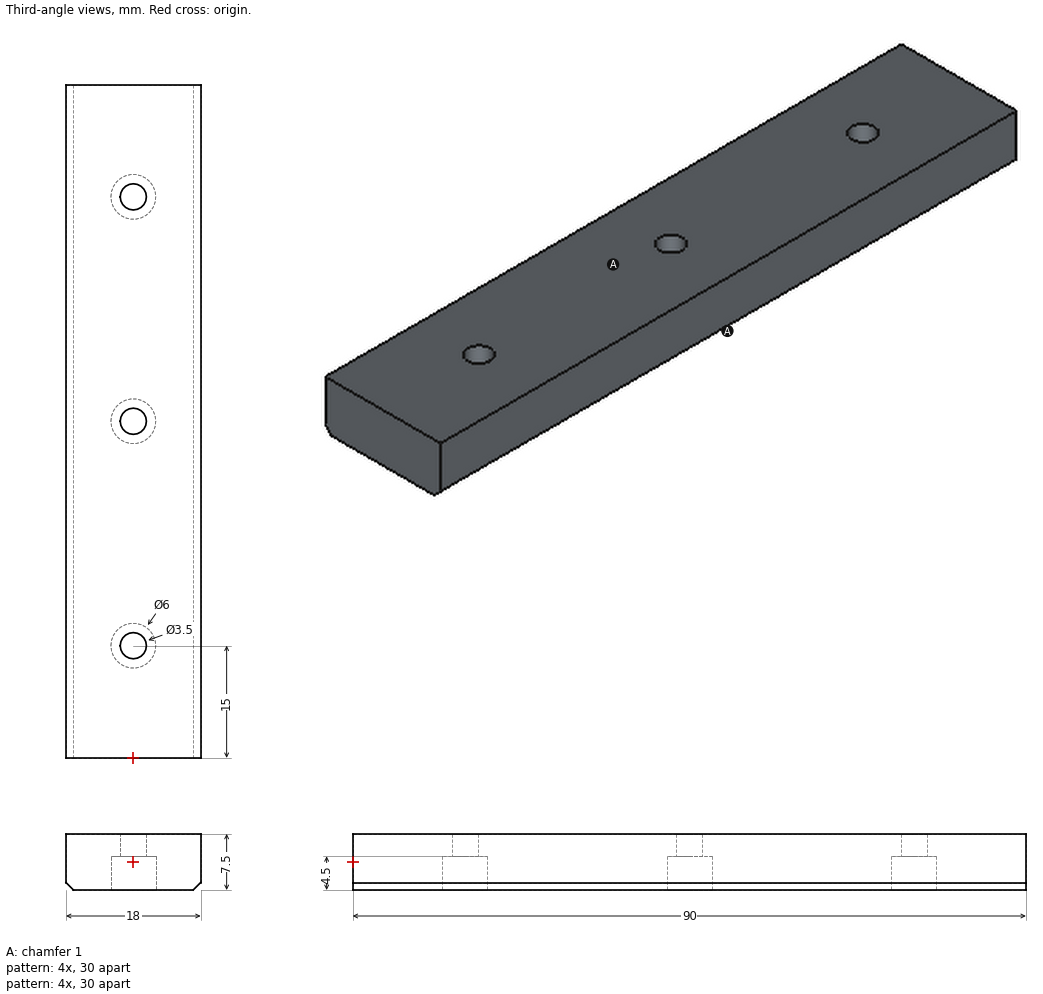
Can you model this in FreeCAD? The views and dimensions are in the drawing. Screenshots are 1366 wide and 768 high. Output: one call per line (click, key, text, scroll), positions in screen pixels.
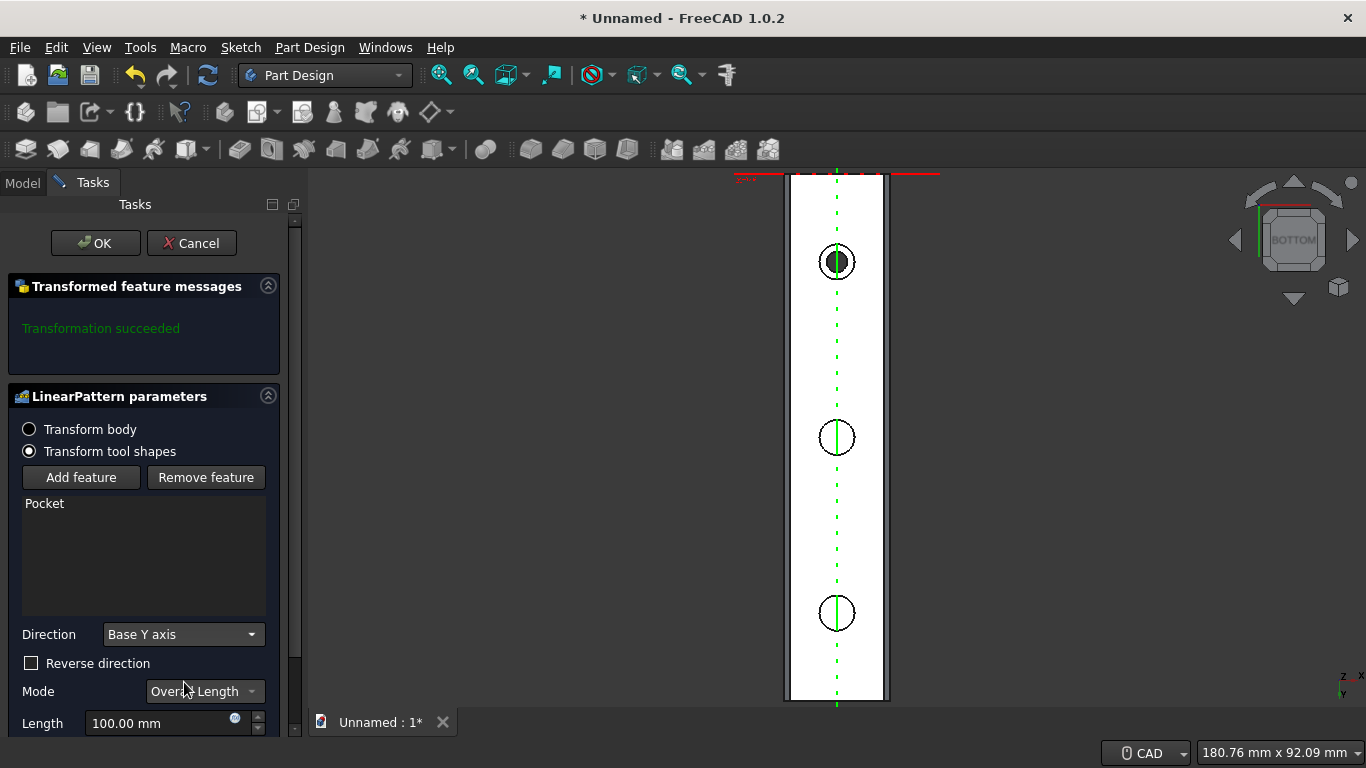
click(206, 692)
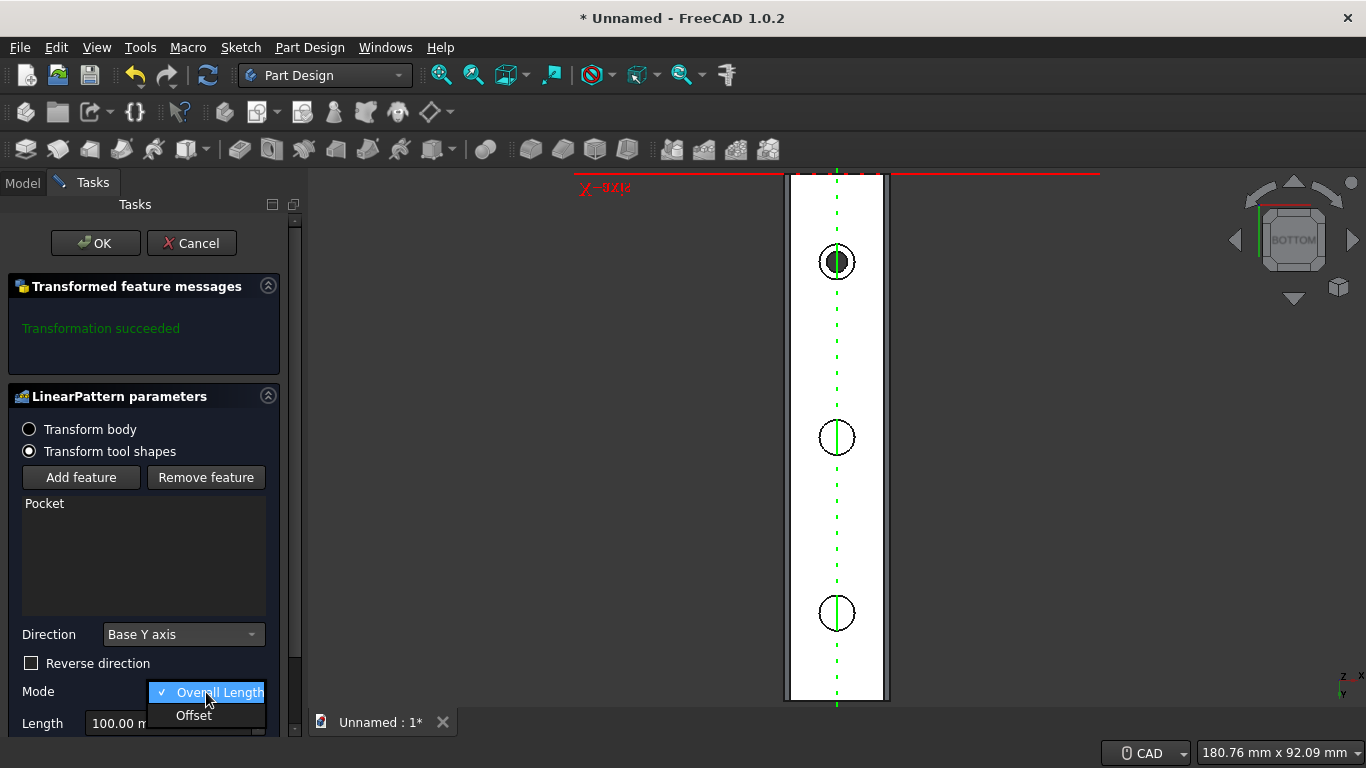
click(206, 716)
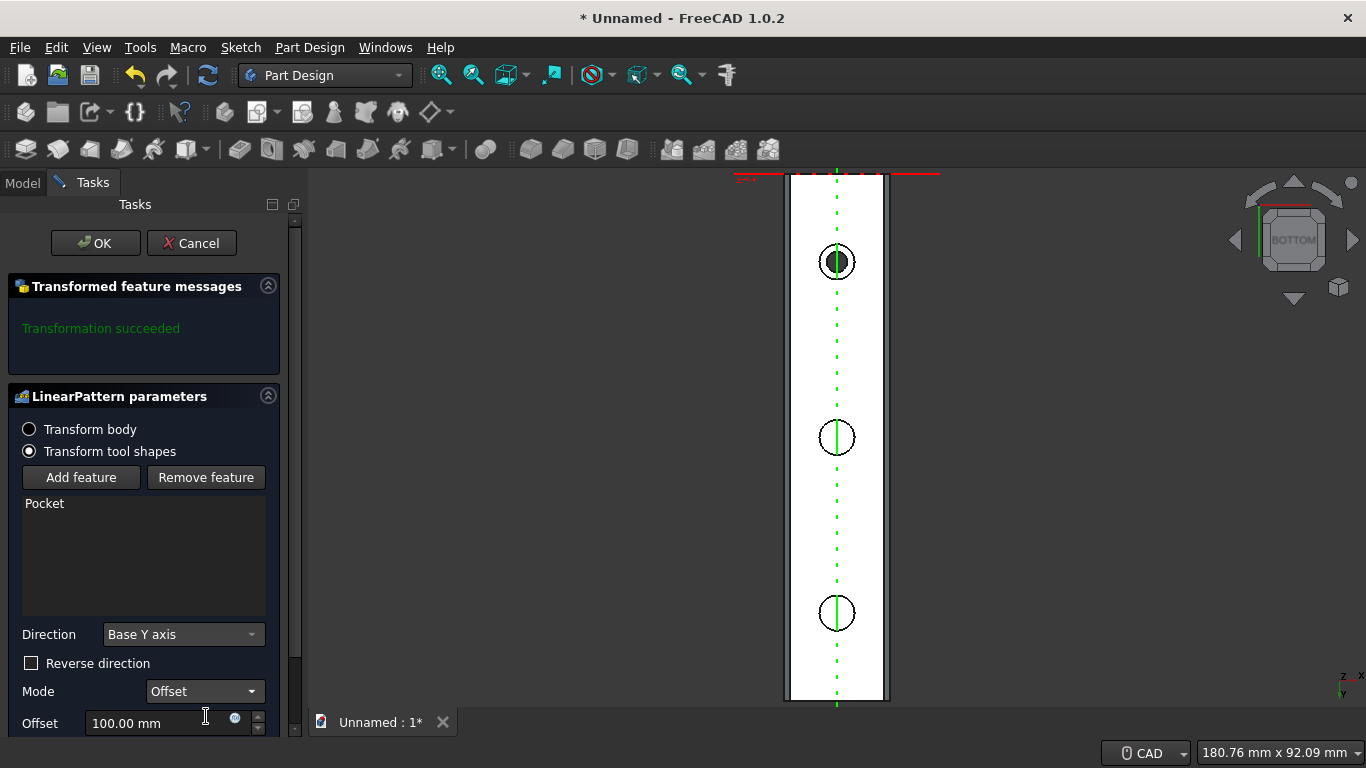
triple_click(168, 723)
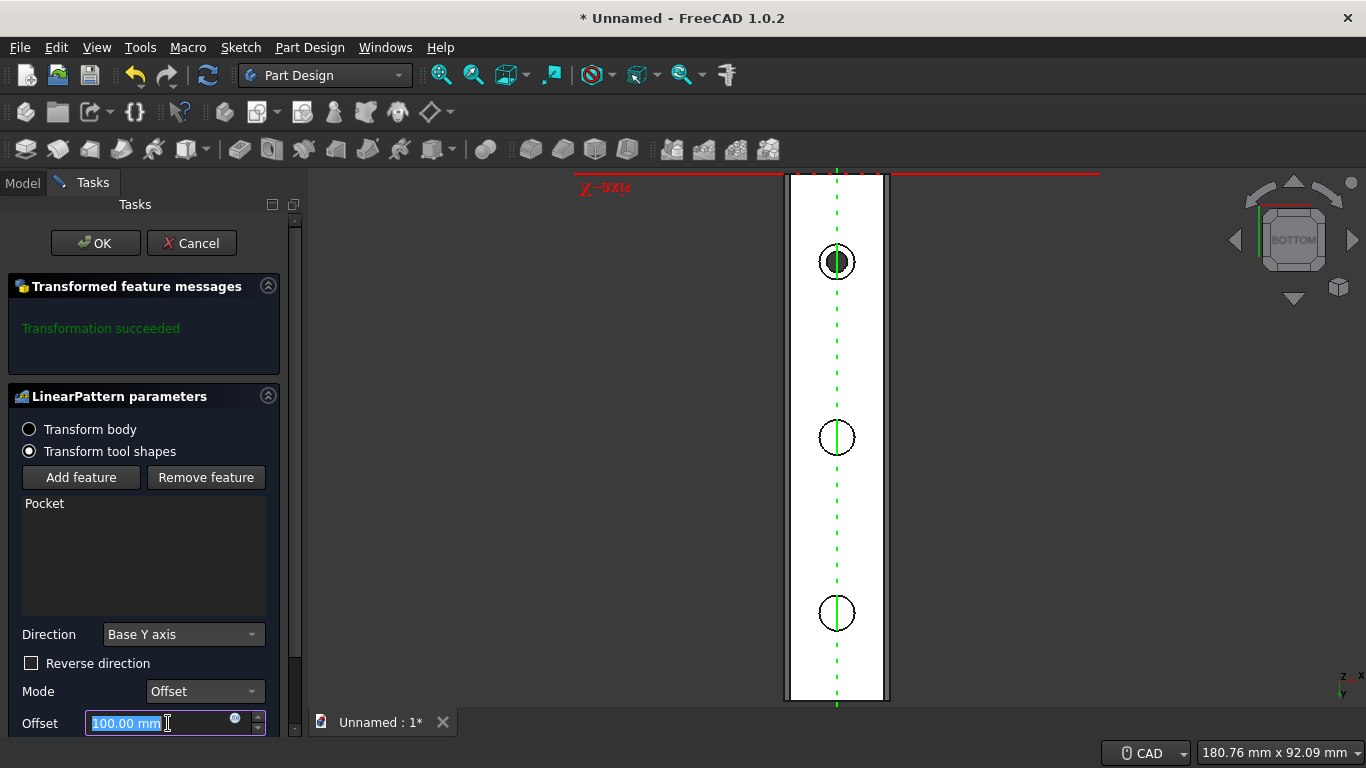
text(30)
key(Tab)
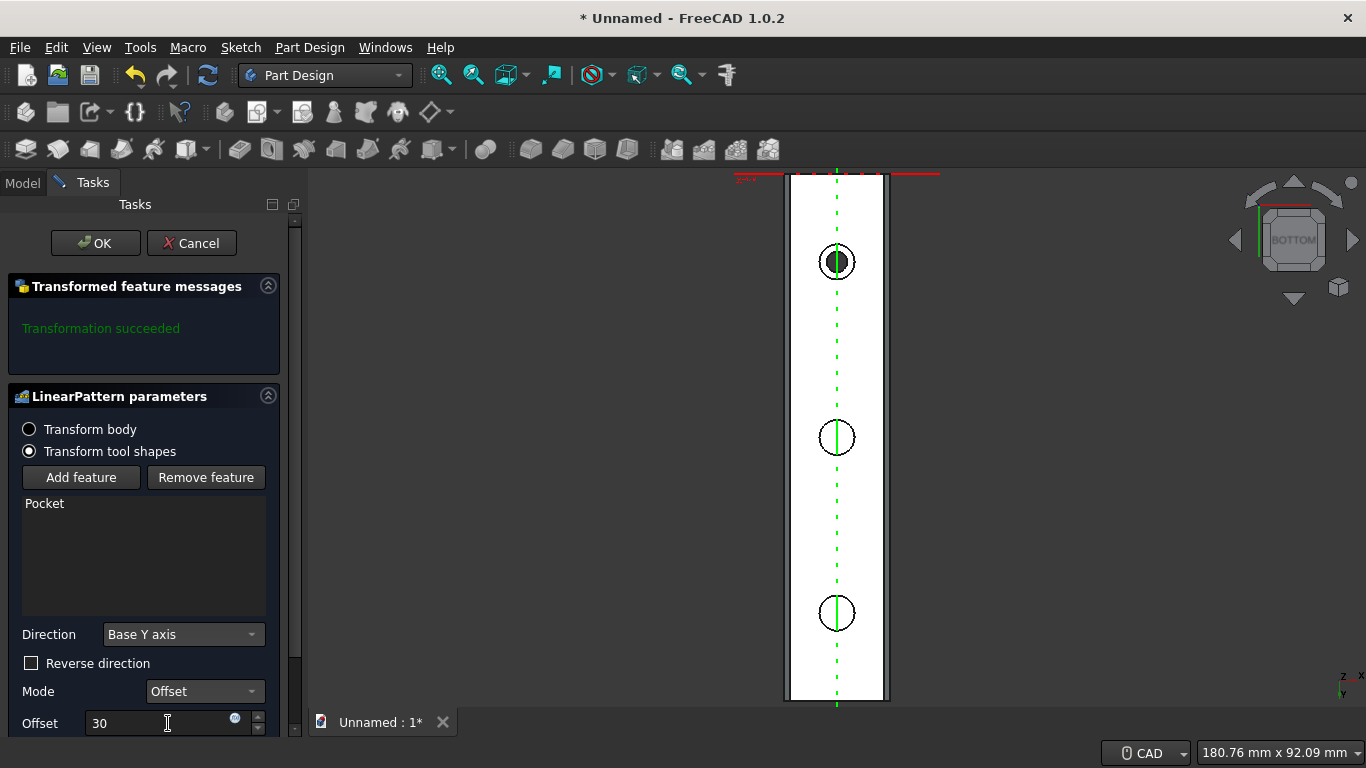
scroll(295, 475, down, 2)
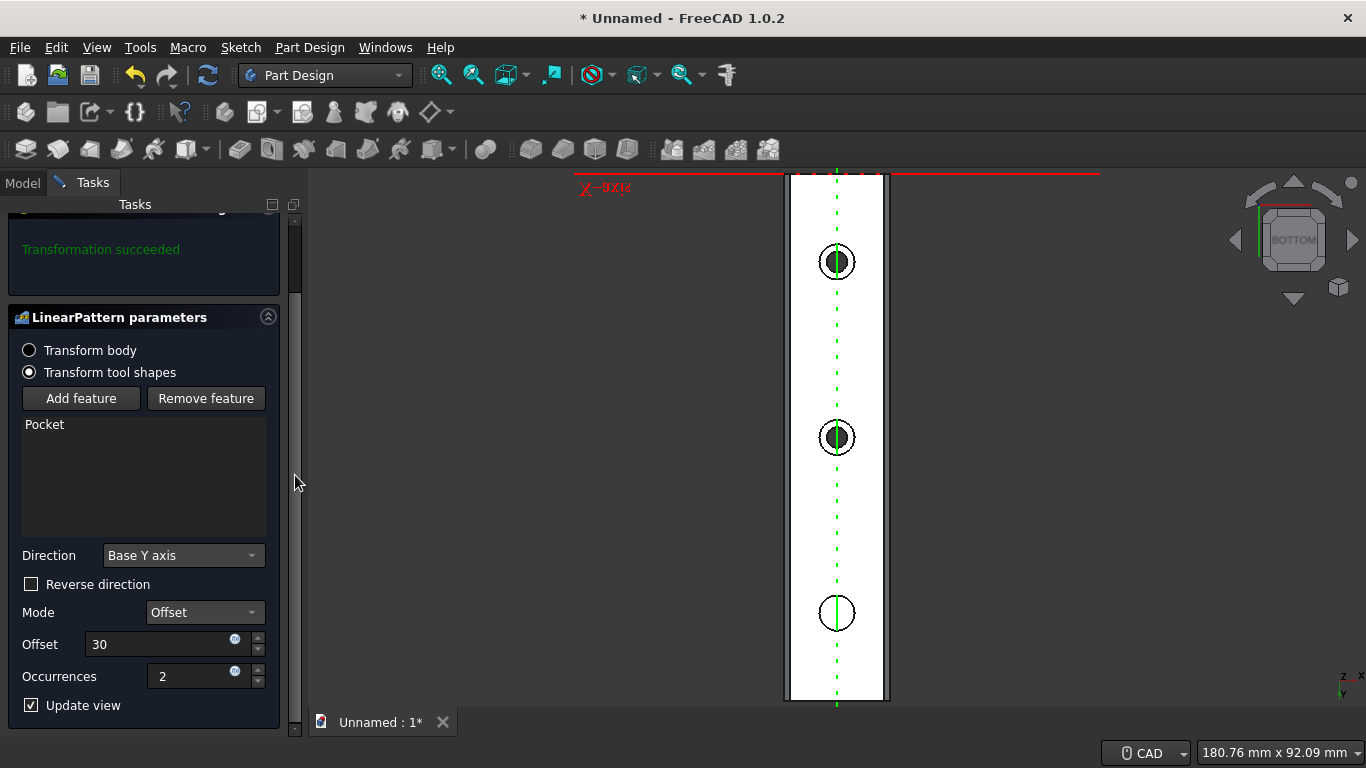
triple_click(198, 676)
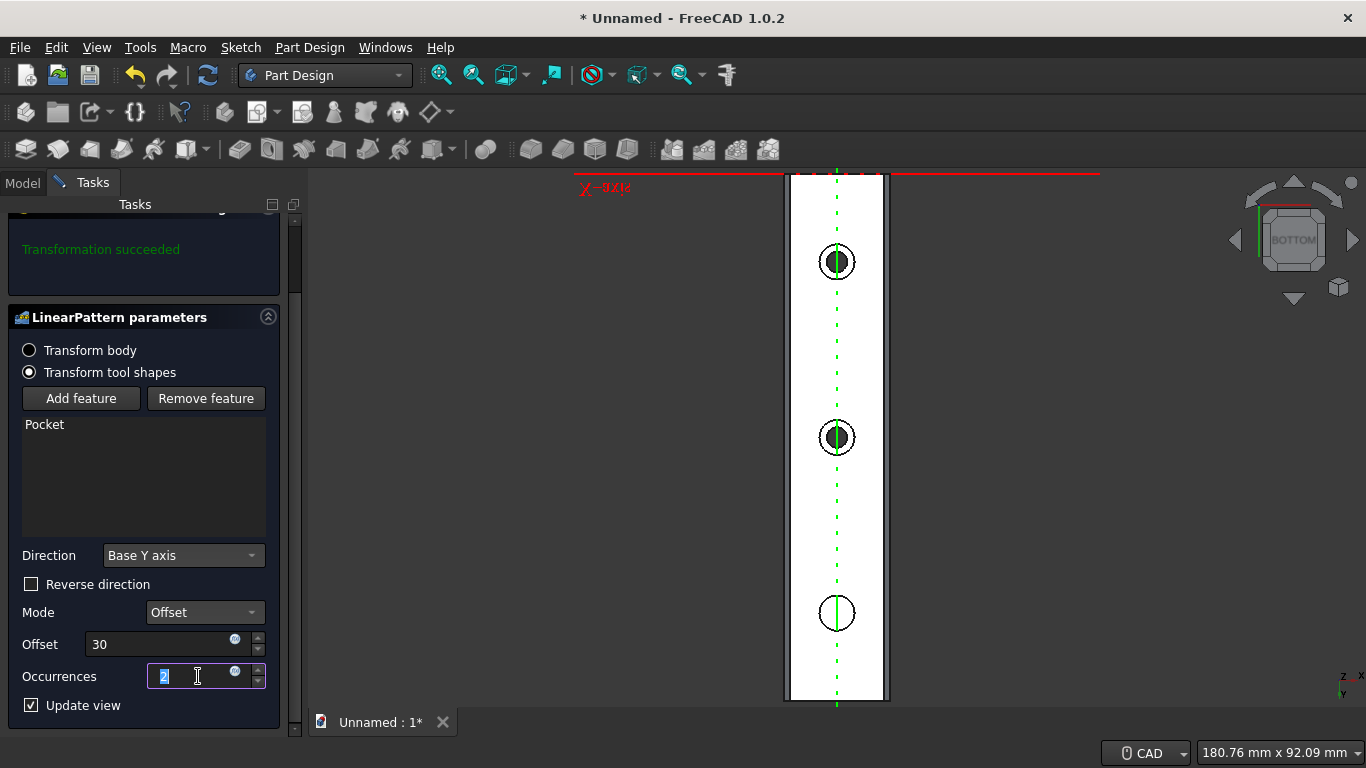
text(4)
key(Tab)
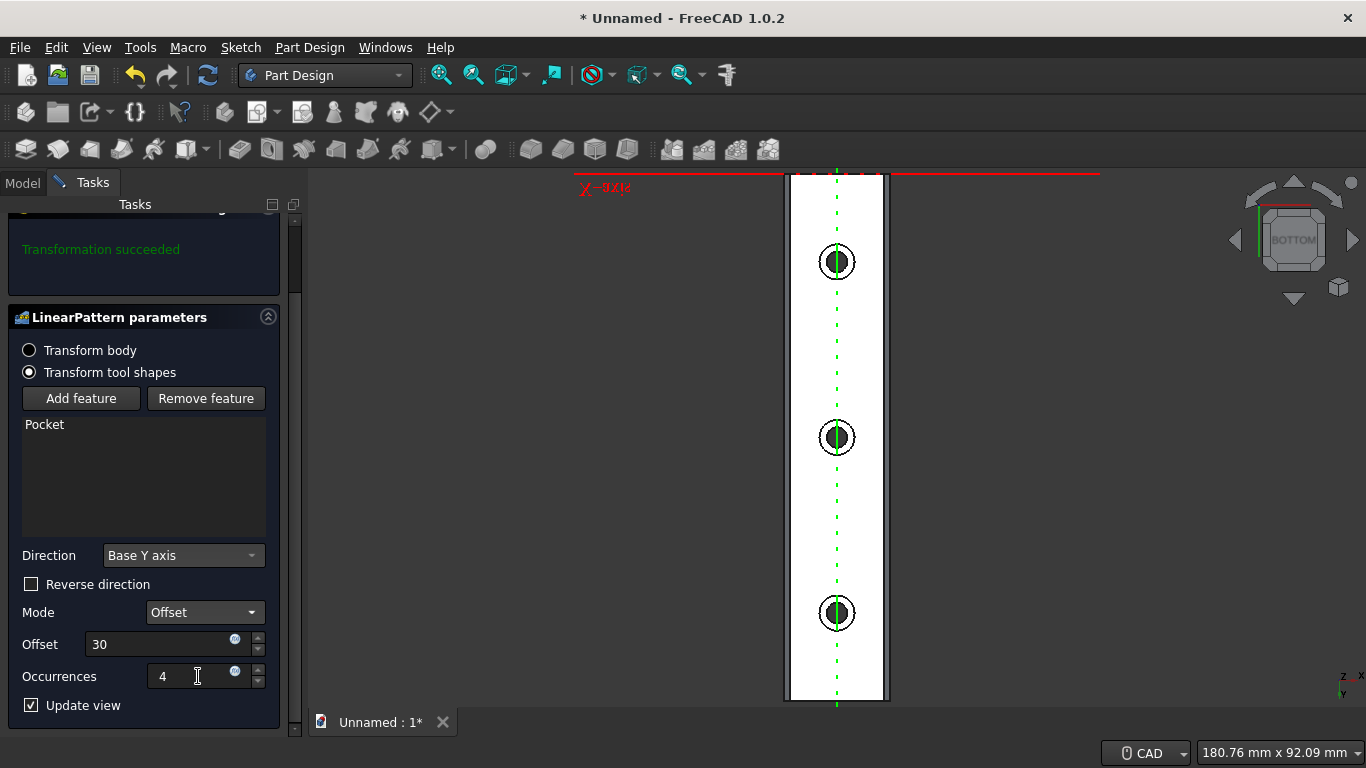
scroll(295, 475, up, 3)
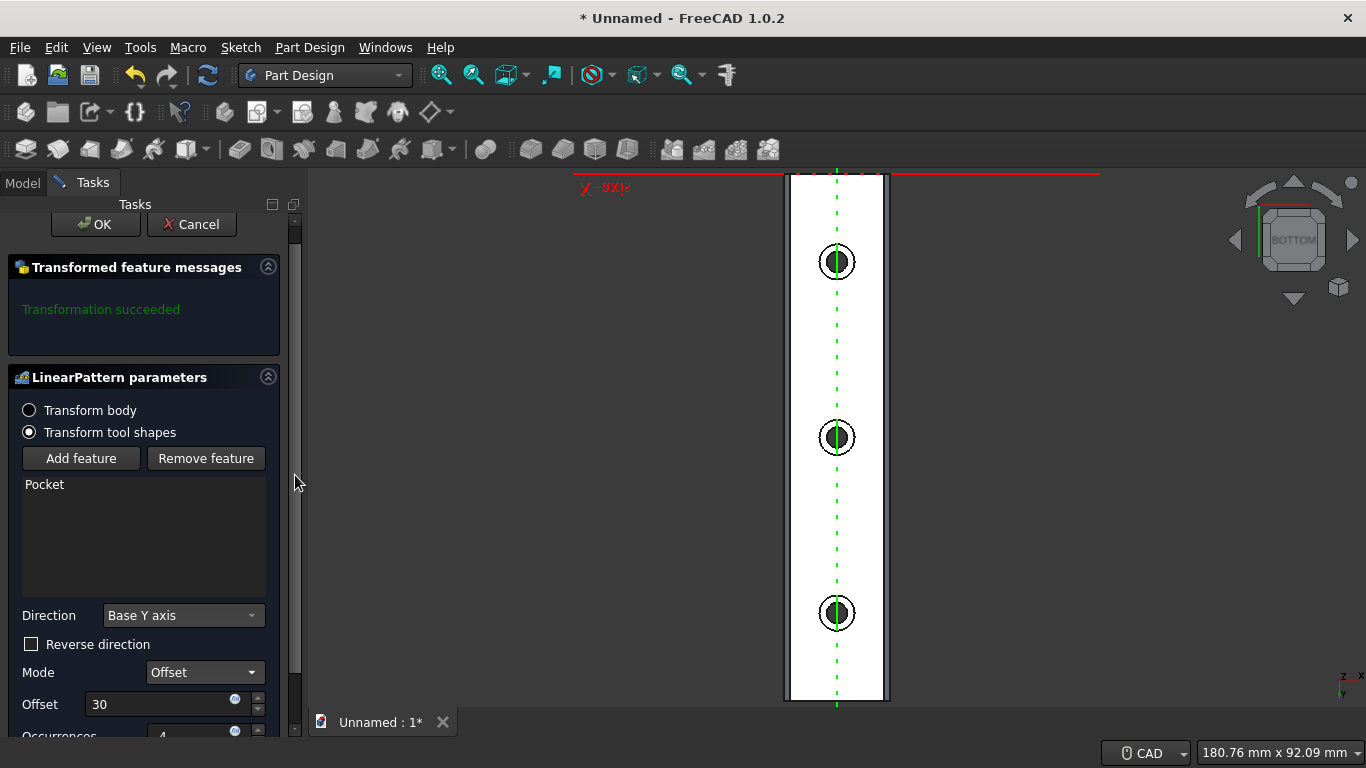
click(96, 243)